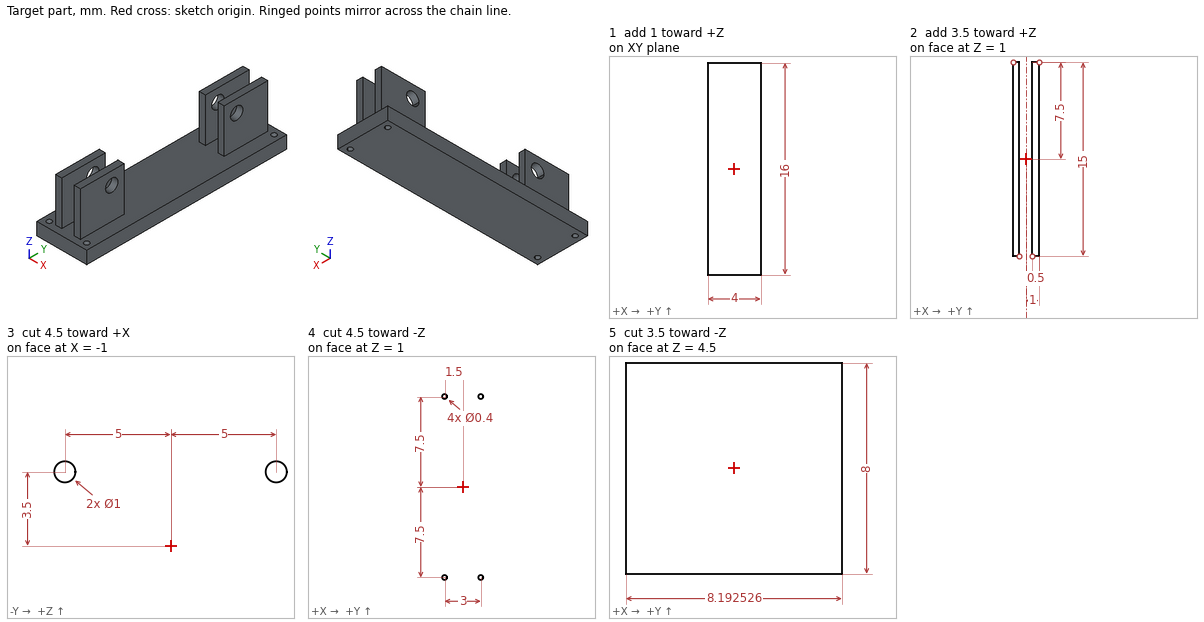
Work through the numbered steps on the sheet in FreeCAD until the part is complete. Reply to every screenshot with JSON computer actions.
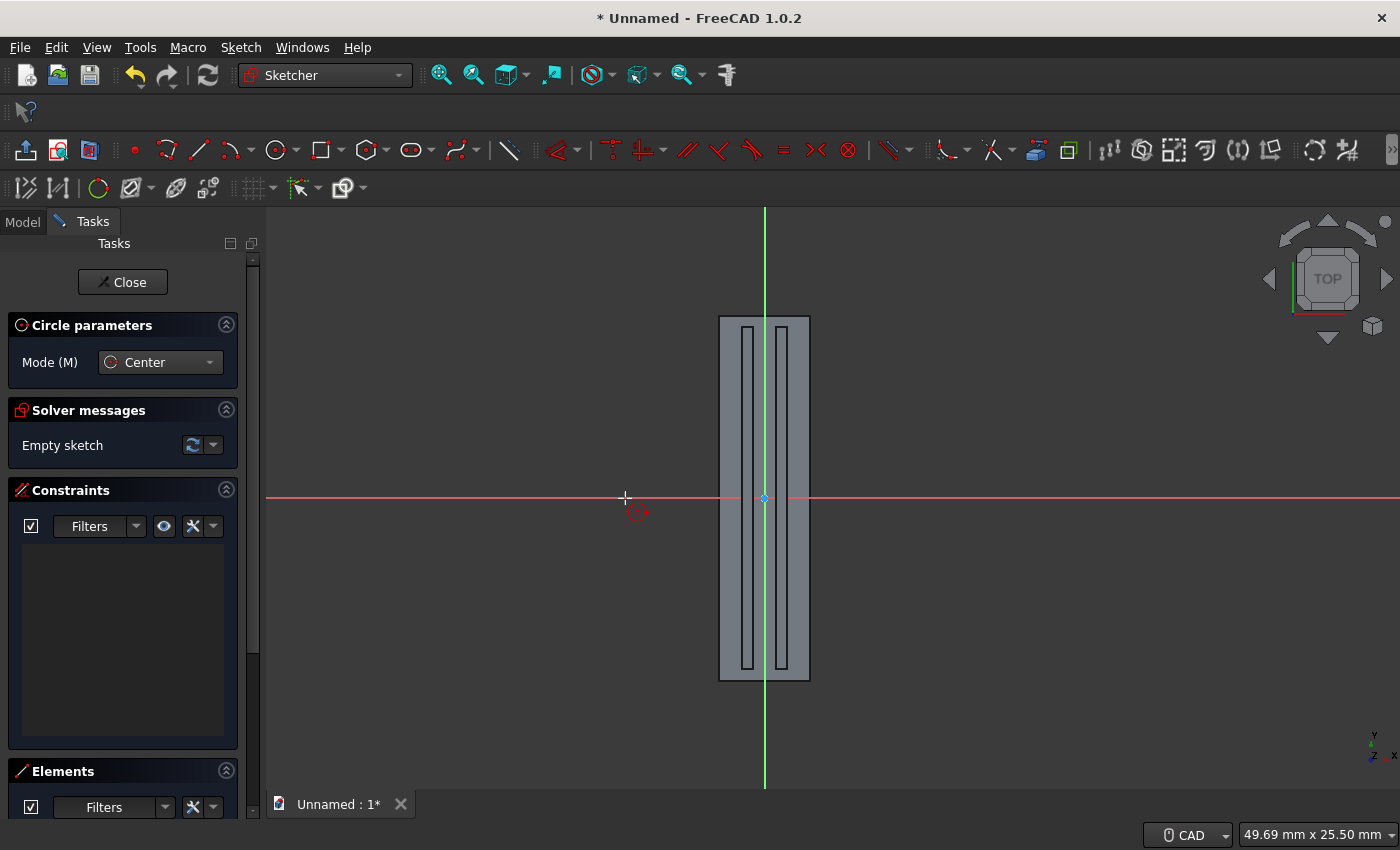
{"action": "scroll", "coordinate": [730, 327], "scroll_direction": "up", "scroll_amount": 9}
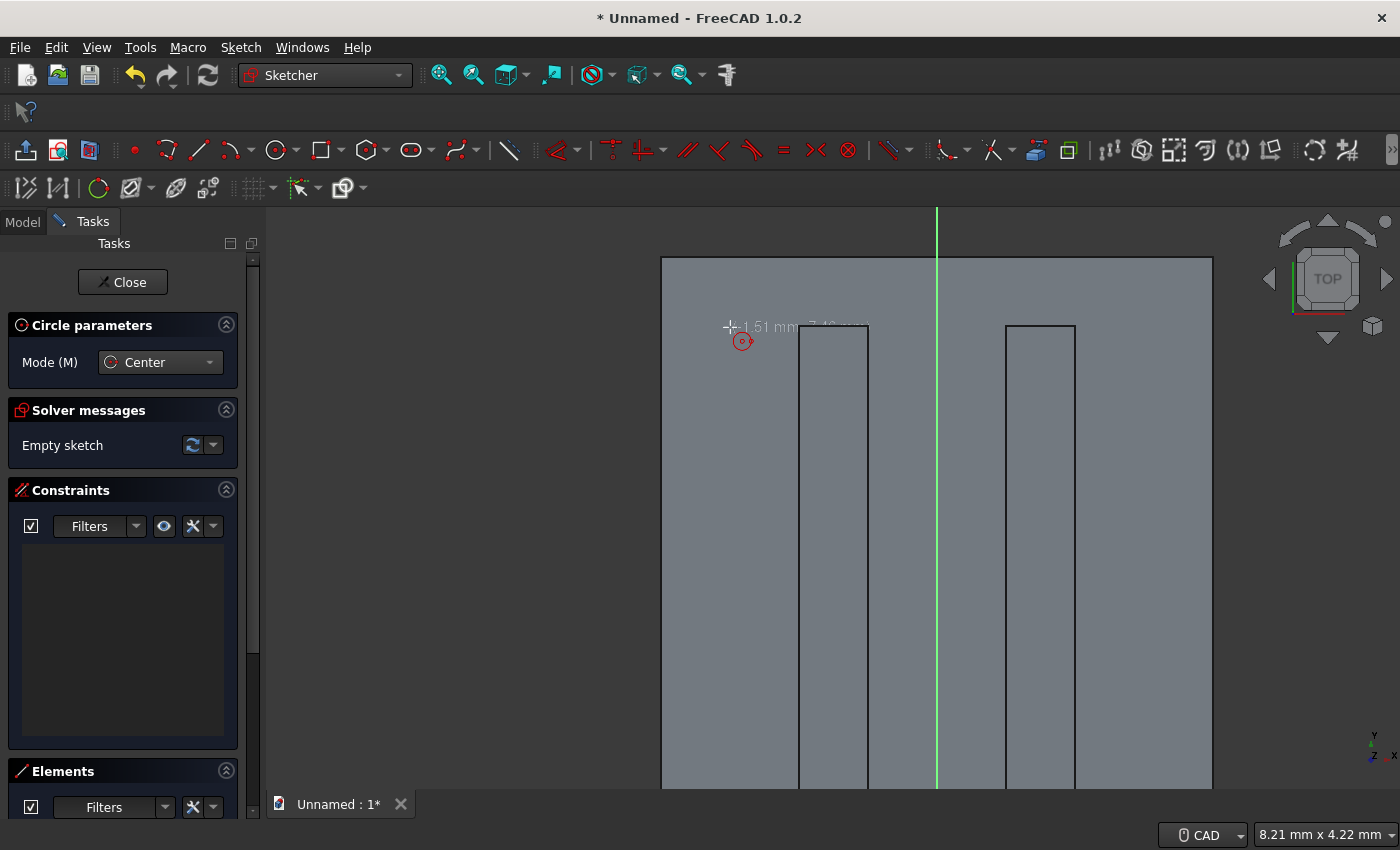
{"action": "scroll", "coordinate": [730, 327], "scroll_direction": "down", "scroll_amount": 9}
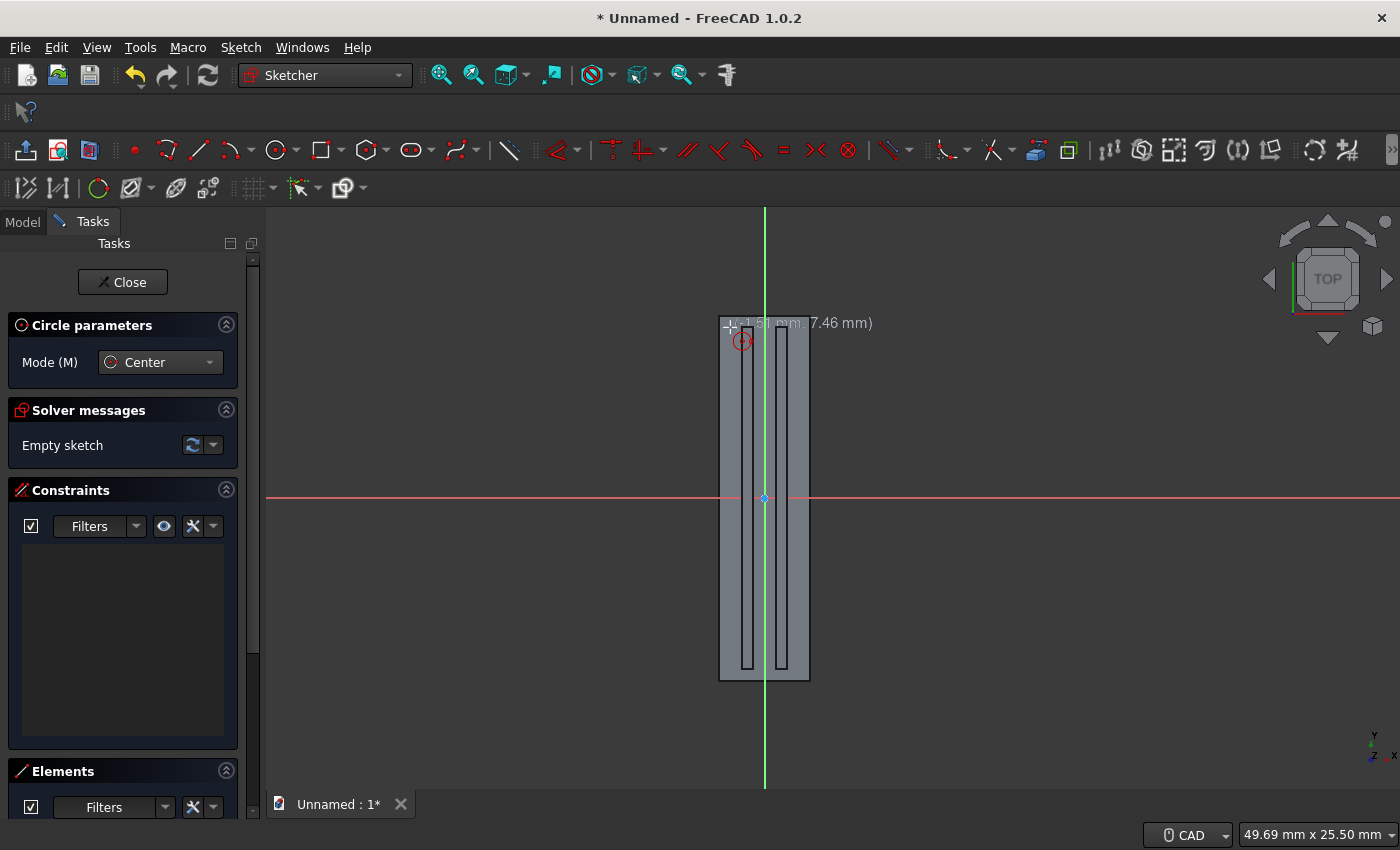
{"action": "left_click", "coordinate": [730, 327]}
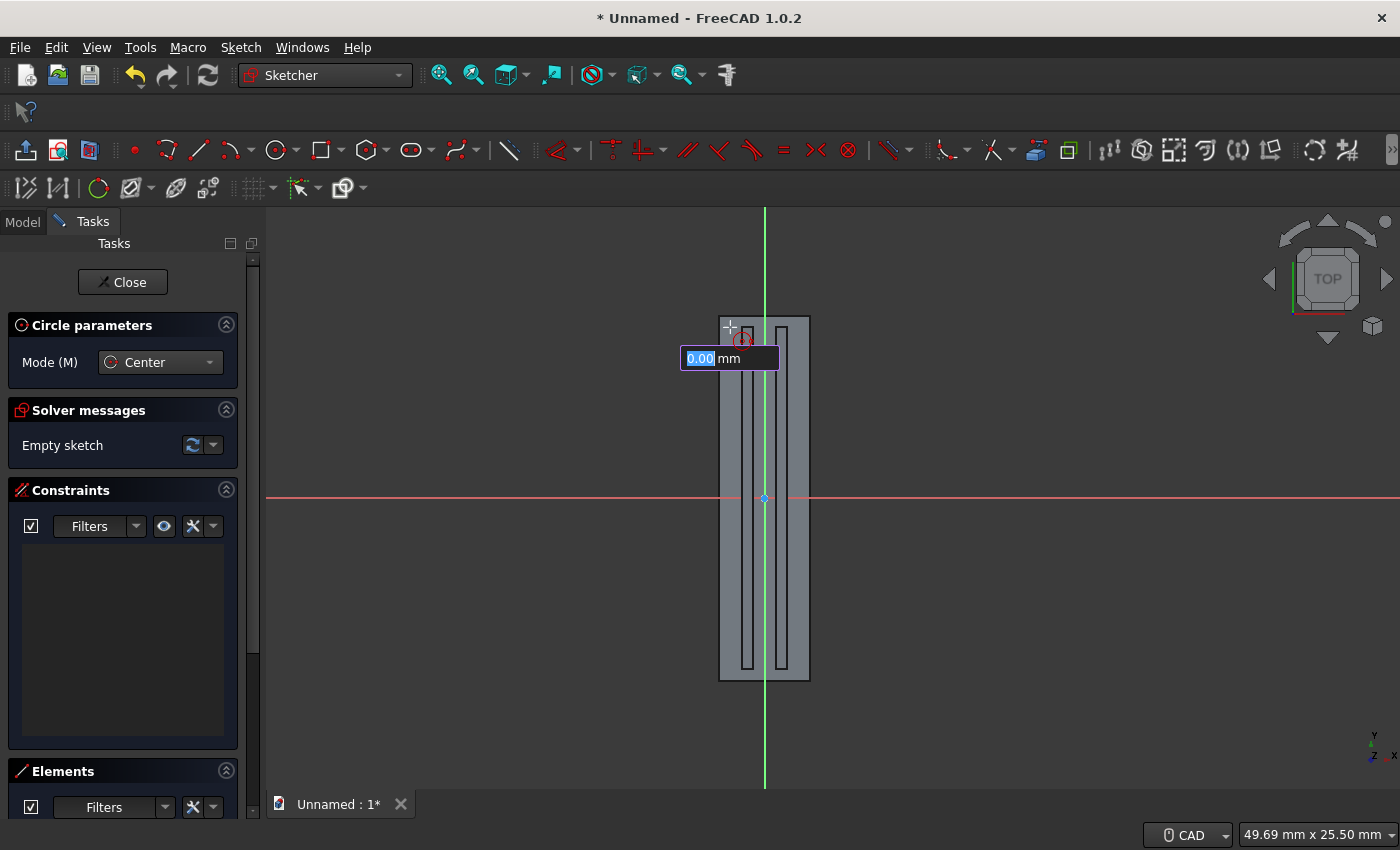
{"action": "scroll", "coordinate": [734, 324], "scroll_direction": "up", "scroll_amount": 7}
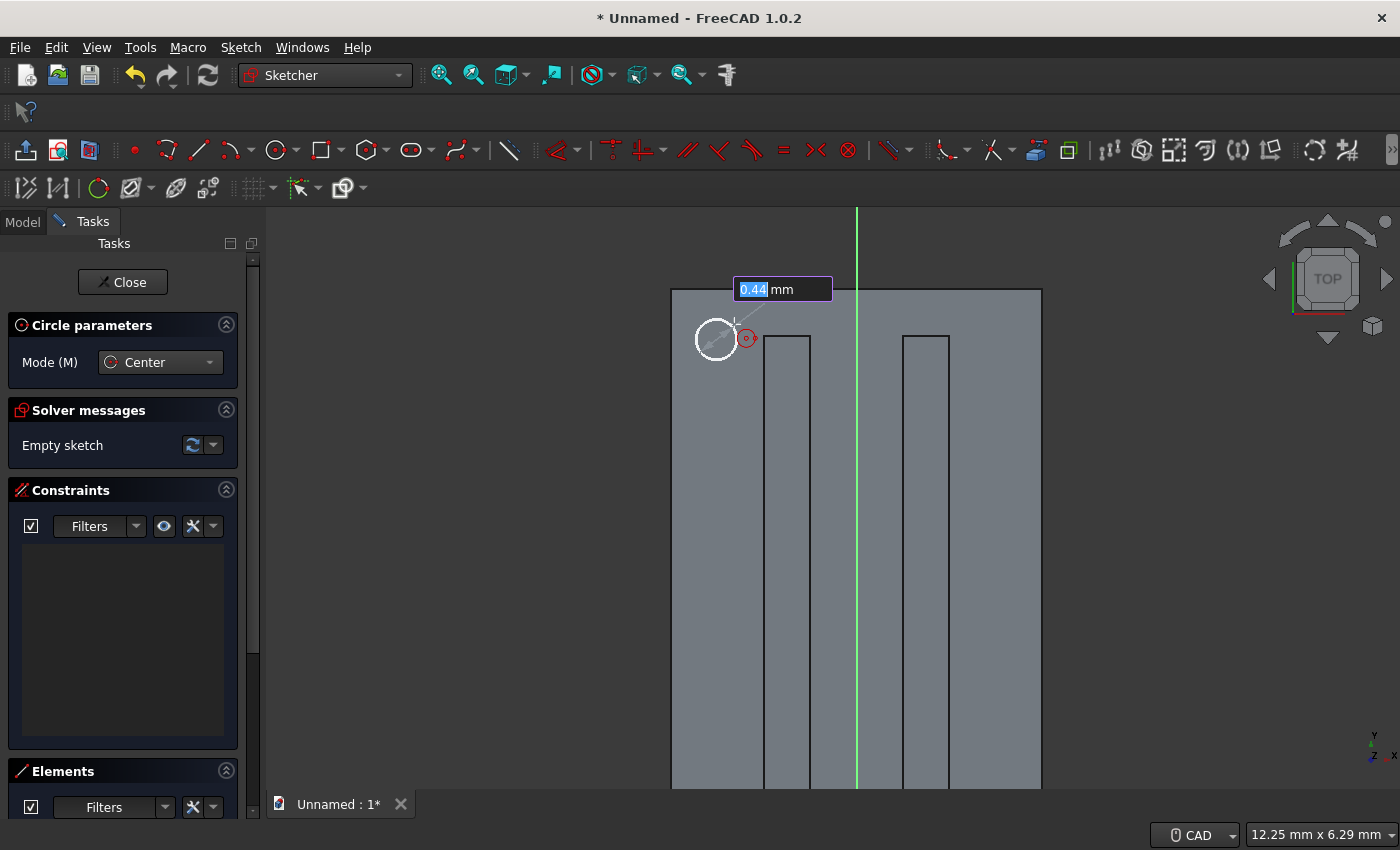
{"action": "left_click", "coordinate": [731, 323]}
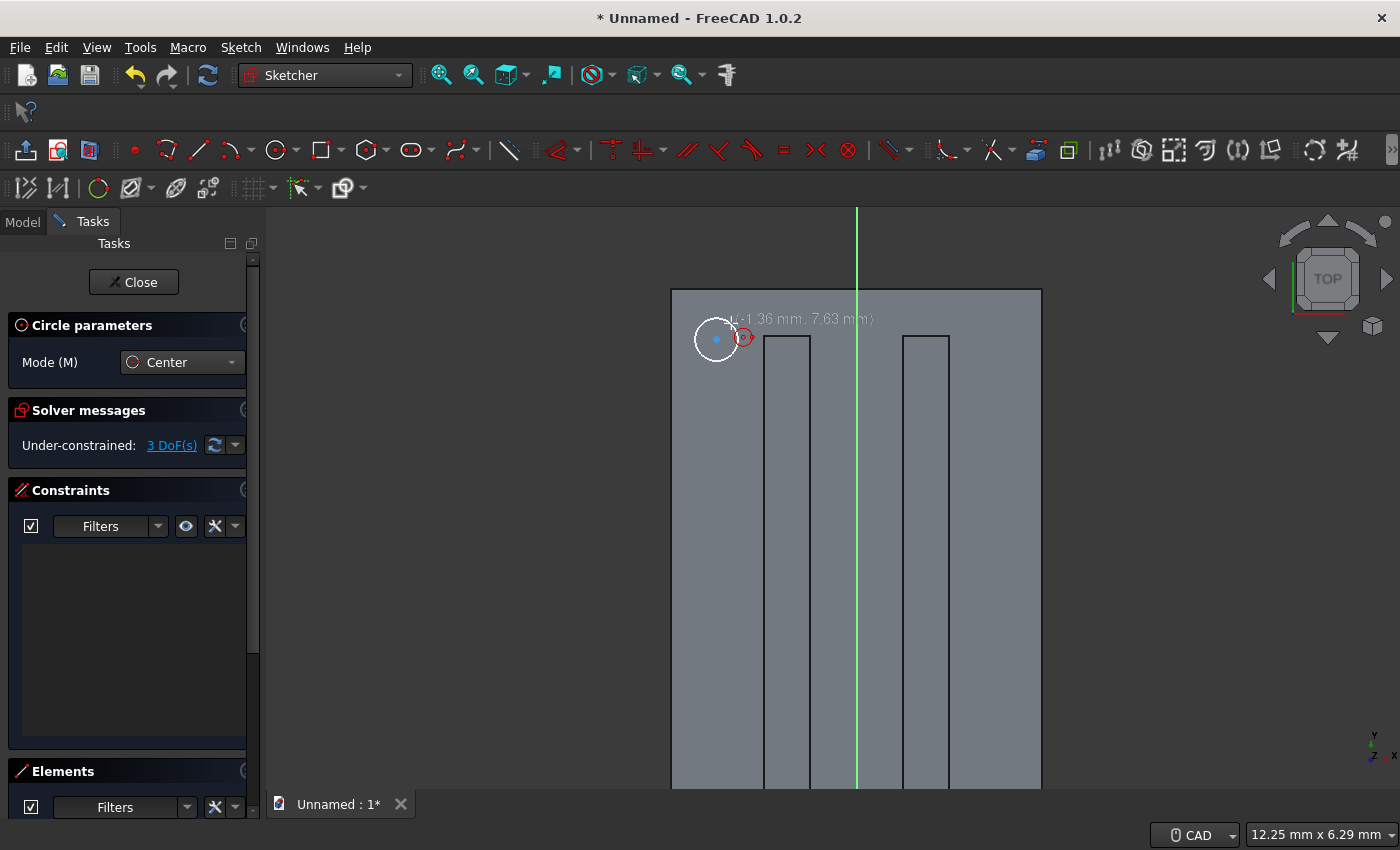
{"action": "scroll", "coordinate": [734, 324], "scroll_direction": "down", "scroll_amount": 7}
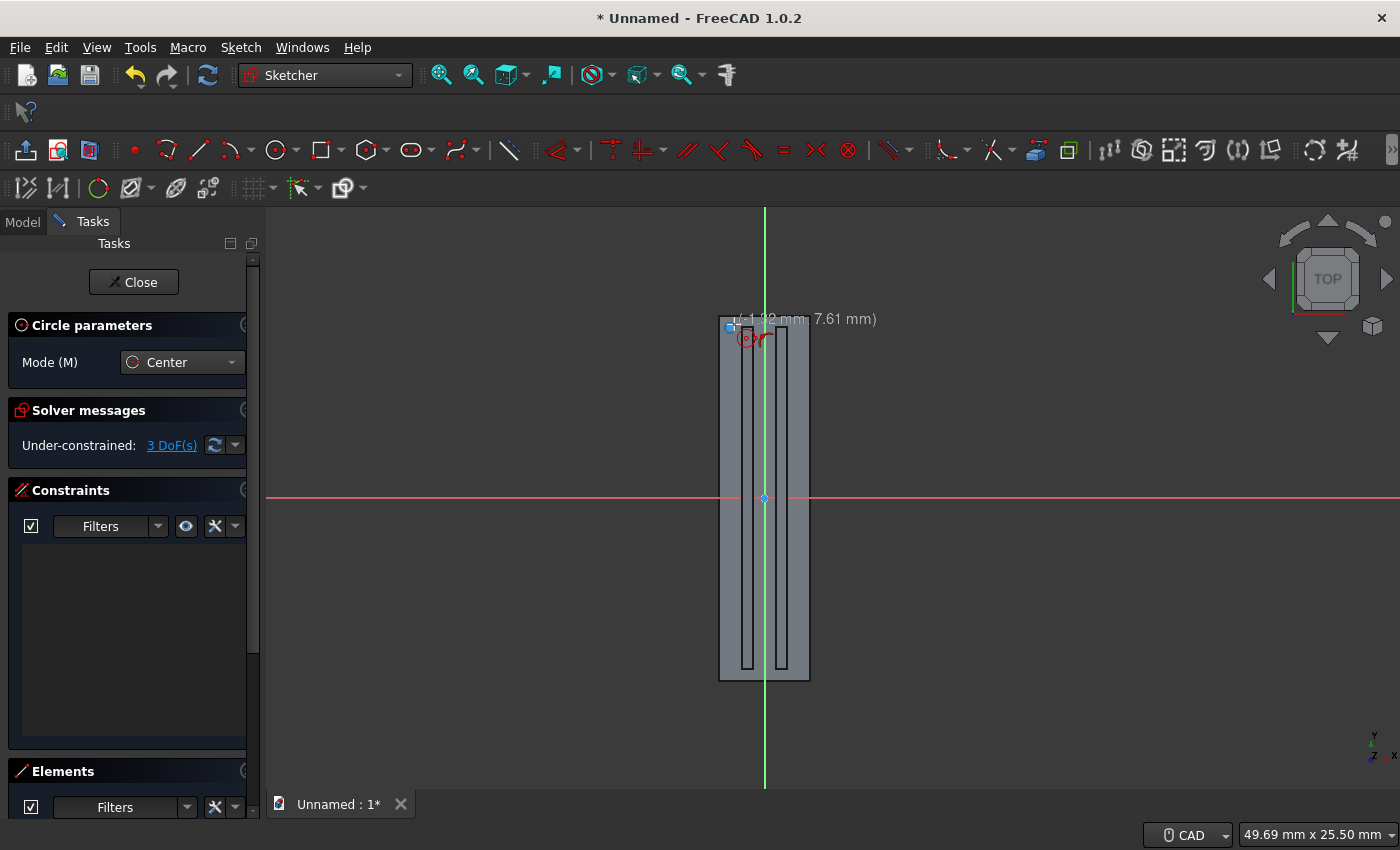
{"action": "scroll", "coordinate": [730, 669], "scroll_direction": "up", "scroll_amount": 9}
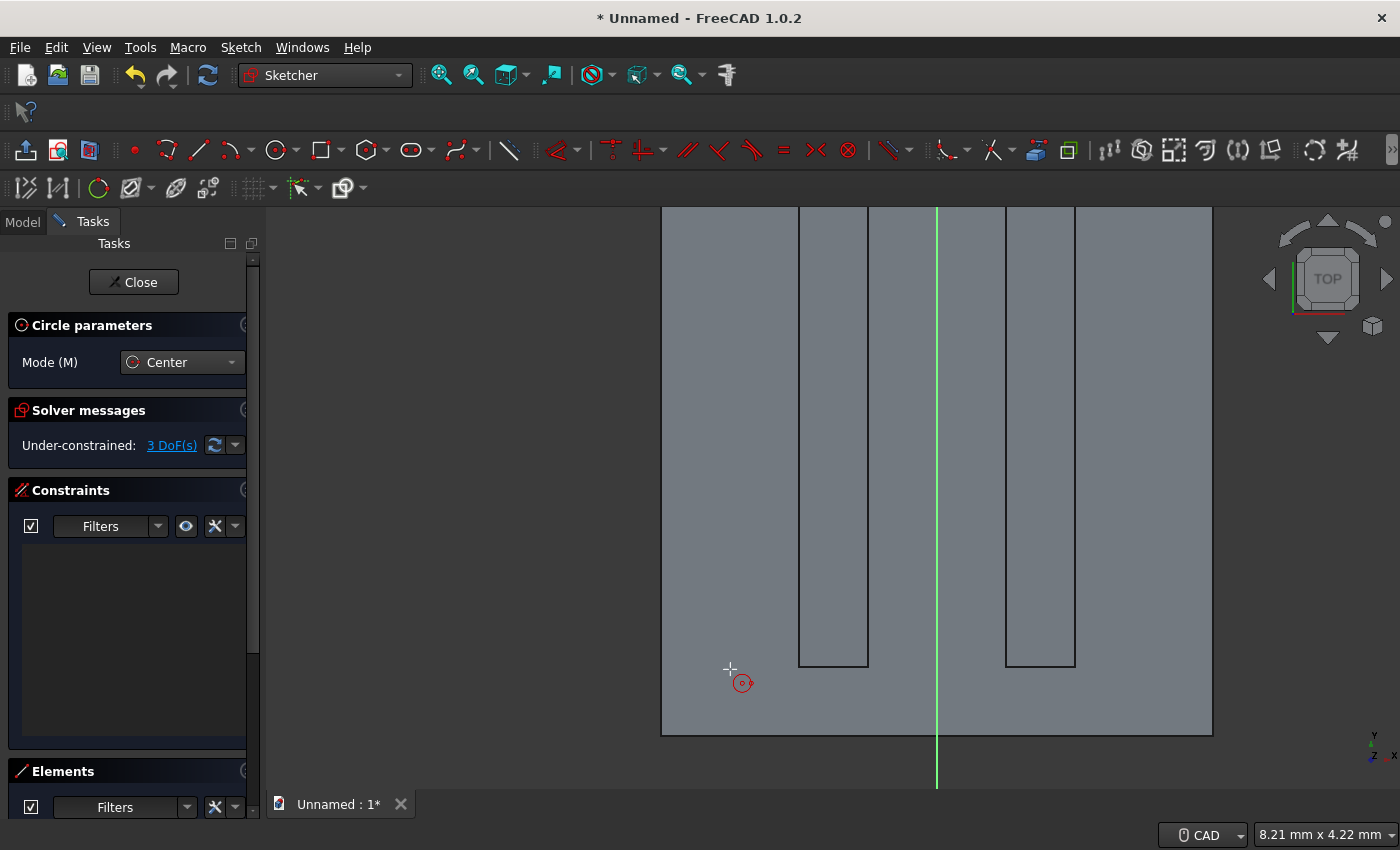
{"action": "scroll", "coordinate": [730, 670], "scroll_direction": "down", "scroll_amount": 9}